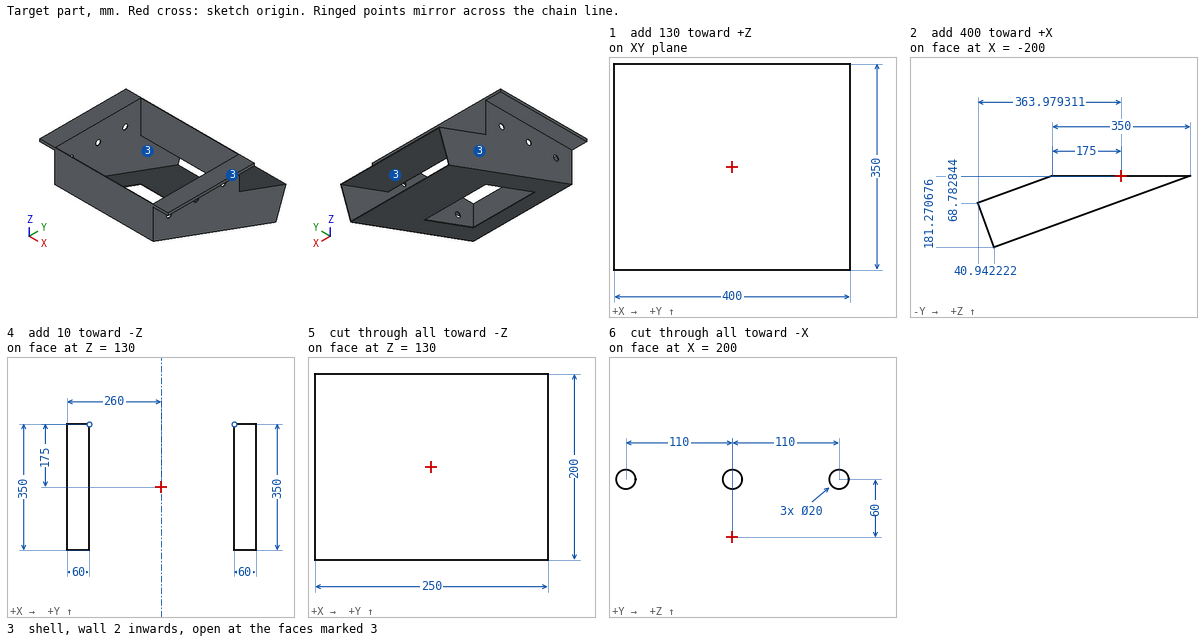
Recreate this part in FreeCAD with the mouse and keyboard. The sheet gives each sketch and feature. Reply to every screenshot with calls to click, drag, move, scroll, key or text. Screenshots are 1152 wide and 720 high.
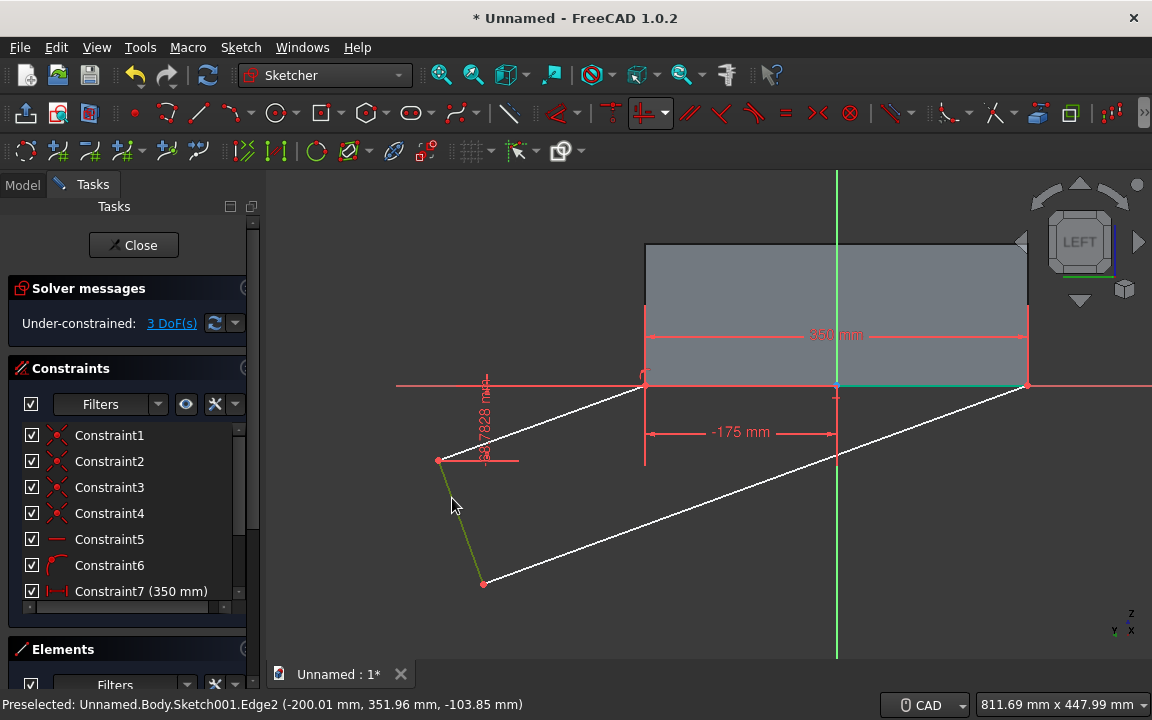
key(l)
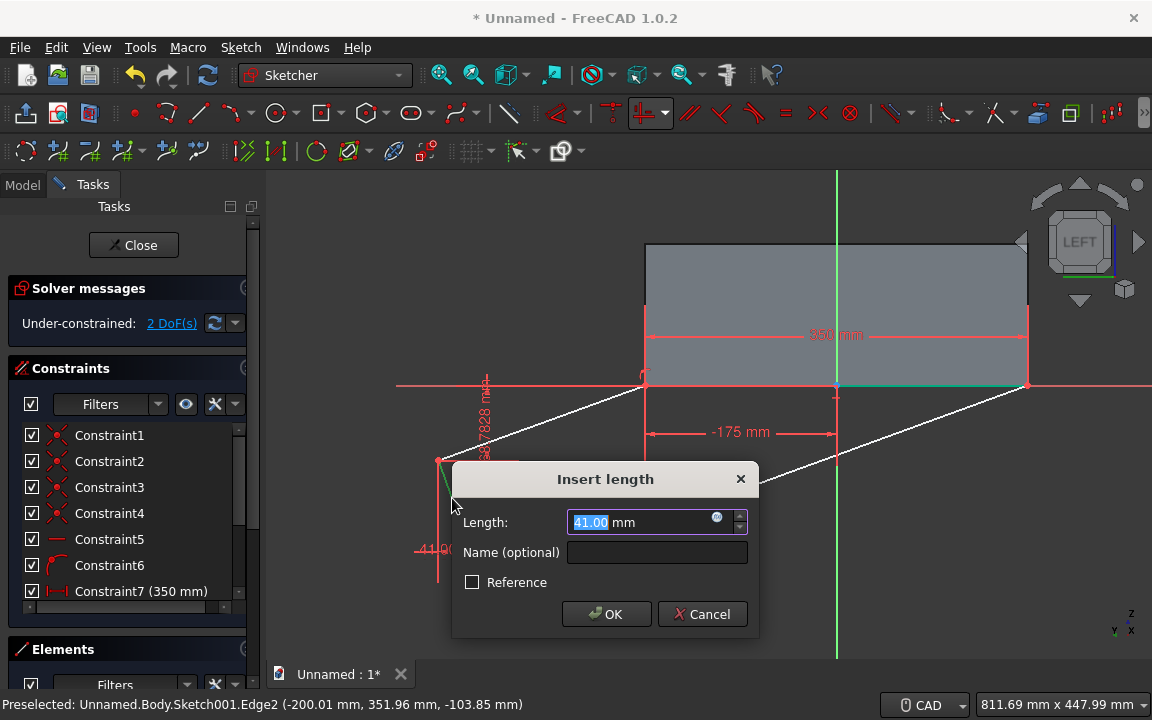
text(40.942222)
key(Return)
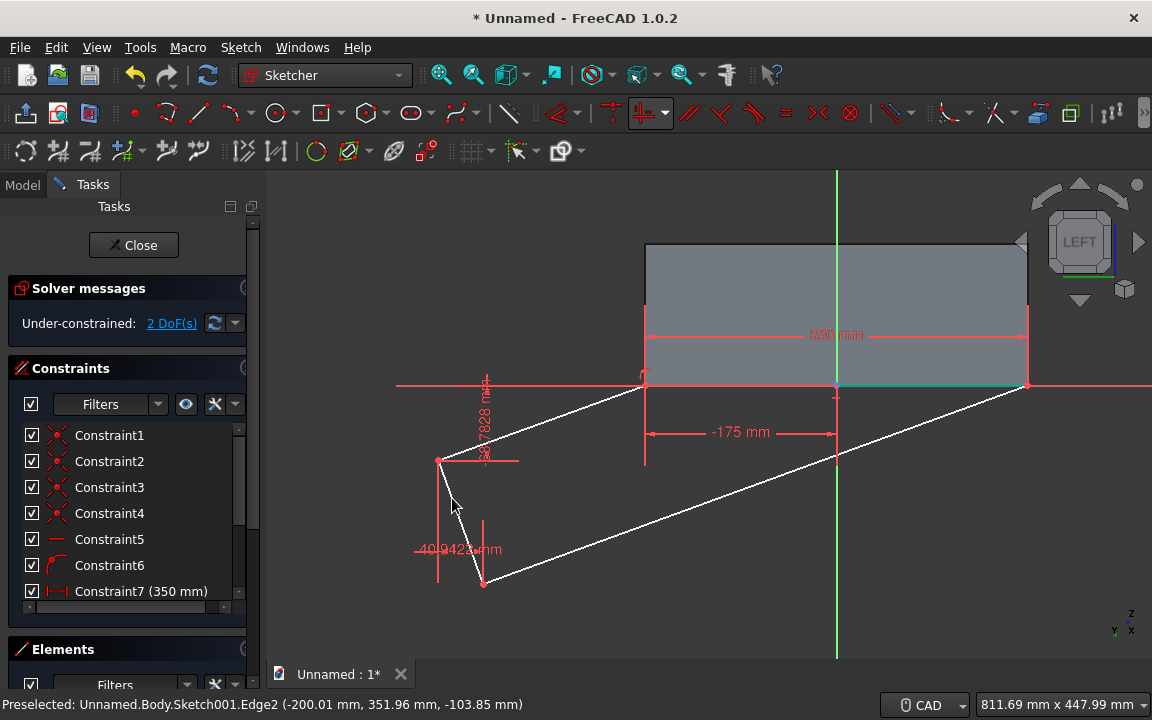
click(438, 461)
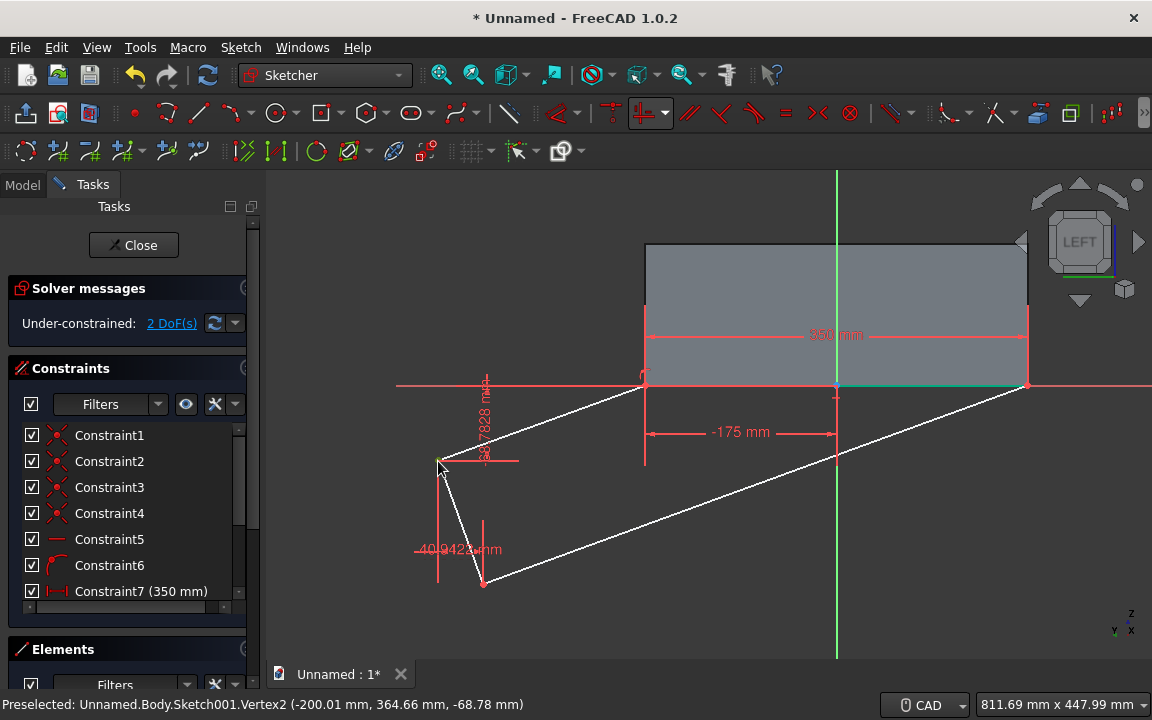
key(l)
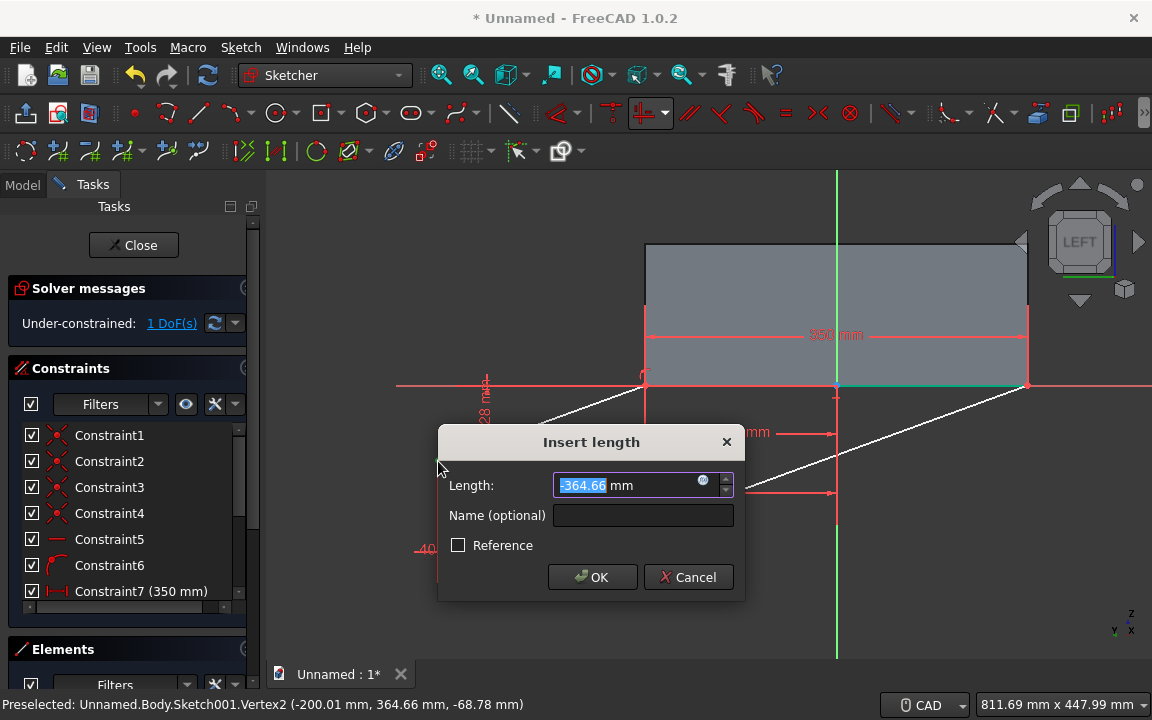
text(-363.979311)
key(Return)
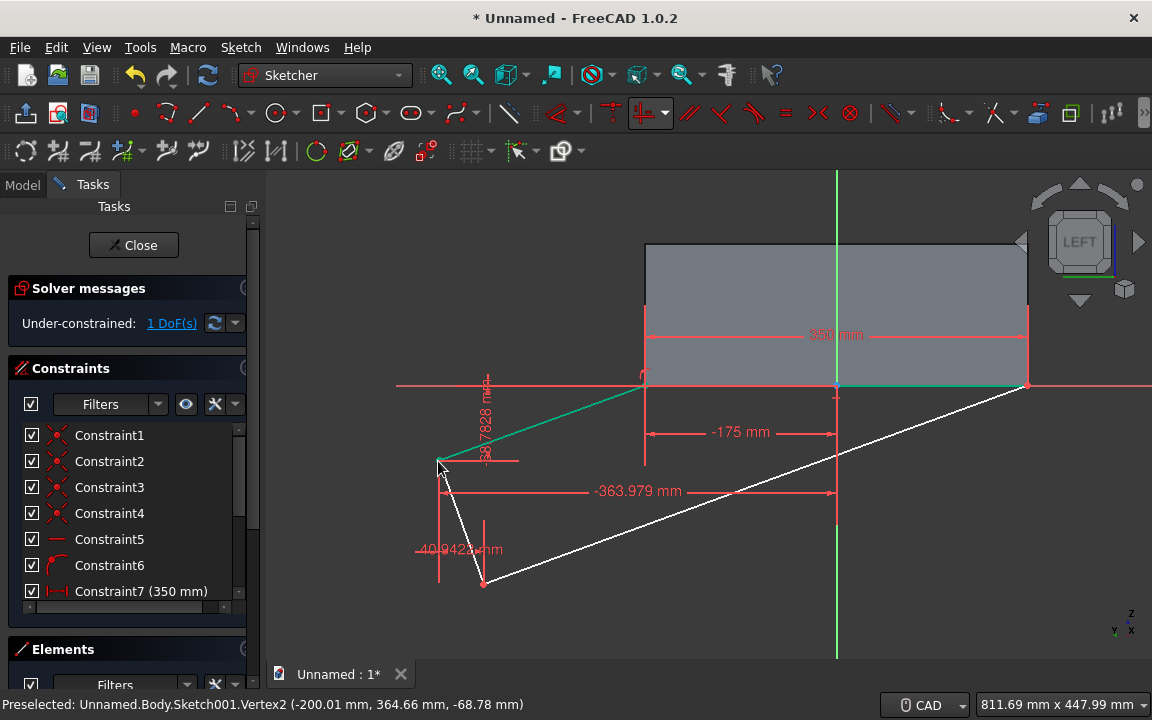
click(484, 584)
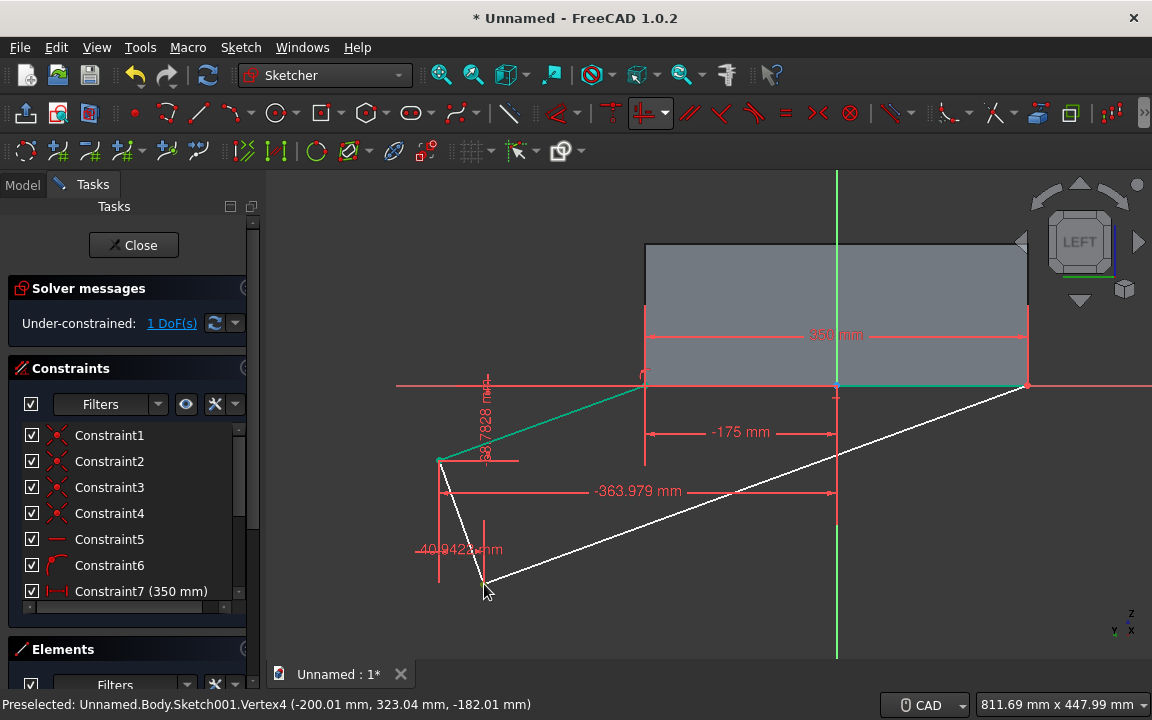
key(i)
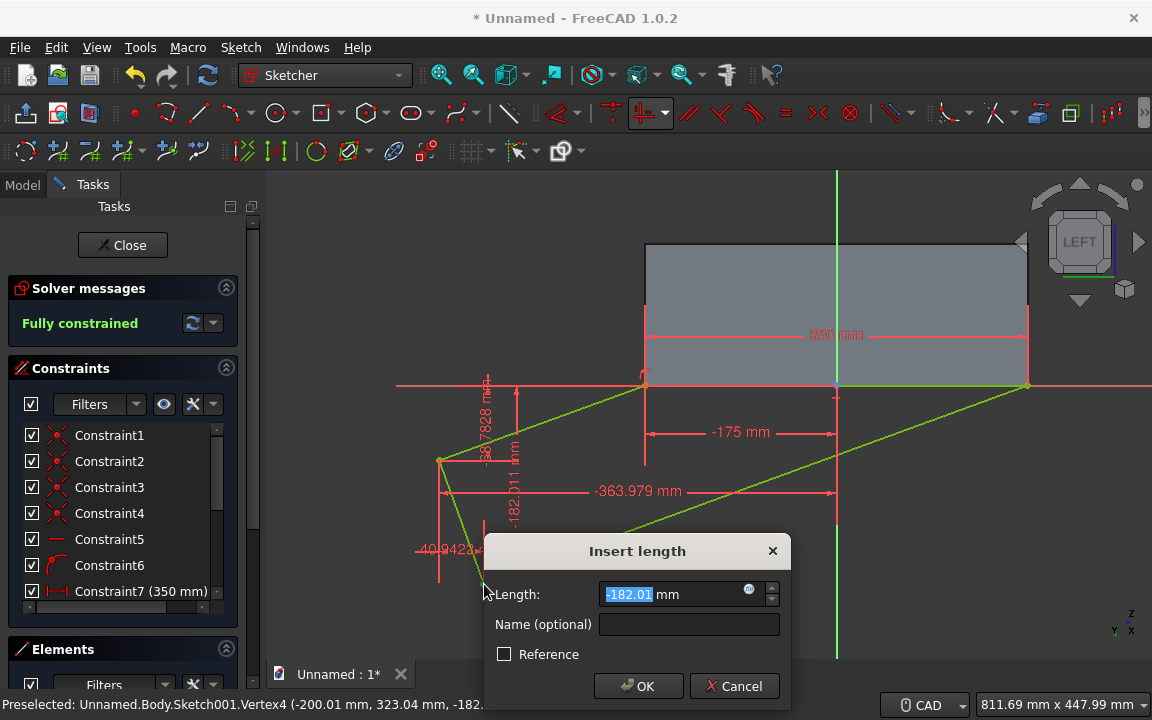
text(-181.270676)
key(Return)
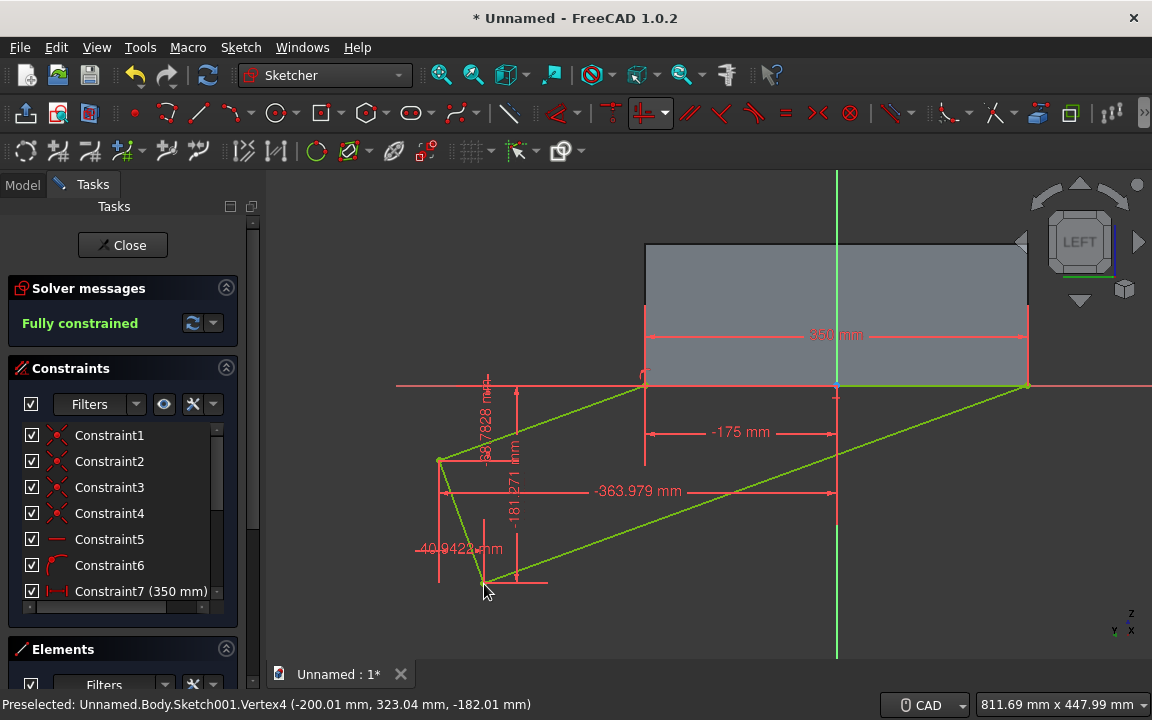
click(123, 245)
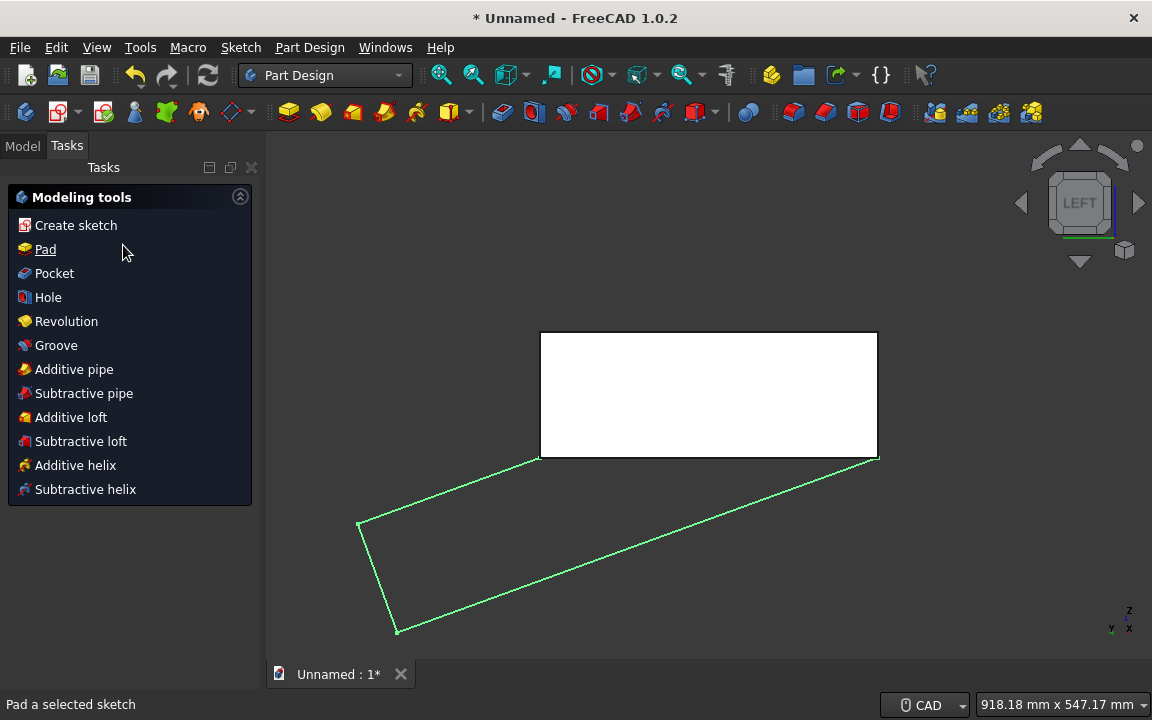
click(290, 112)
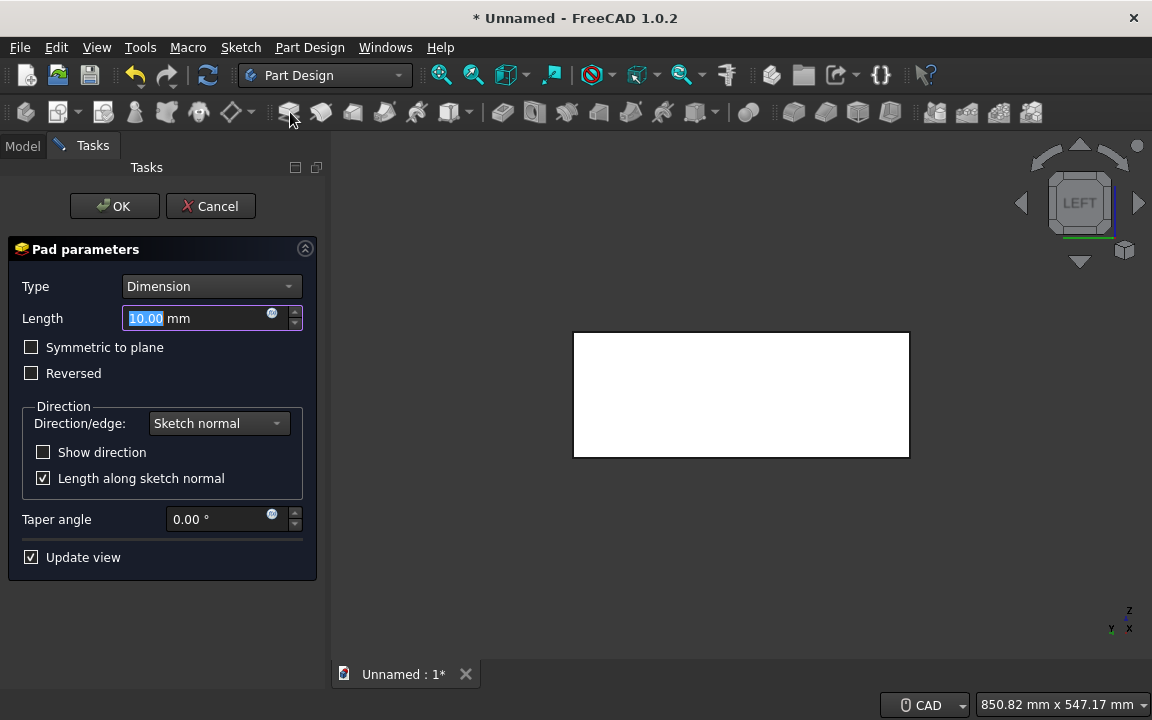
text(400)
key(Tab)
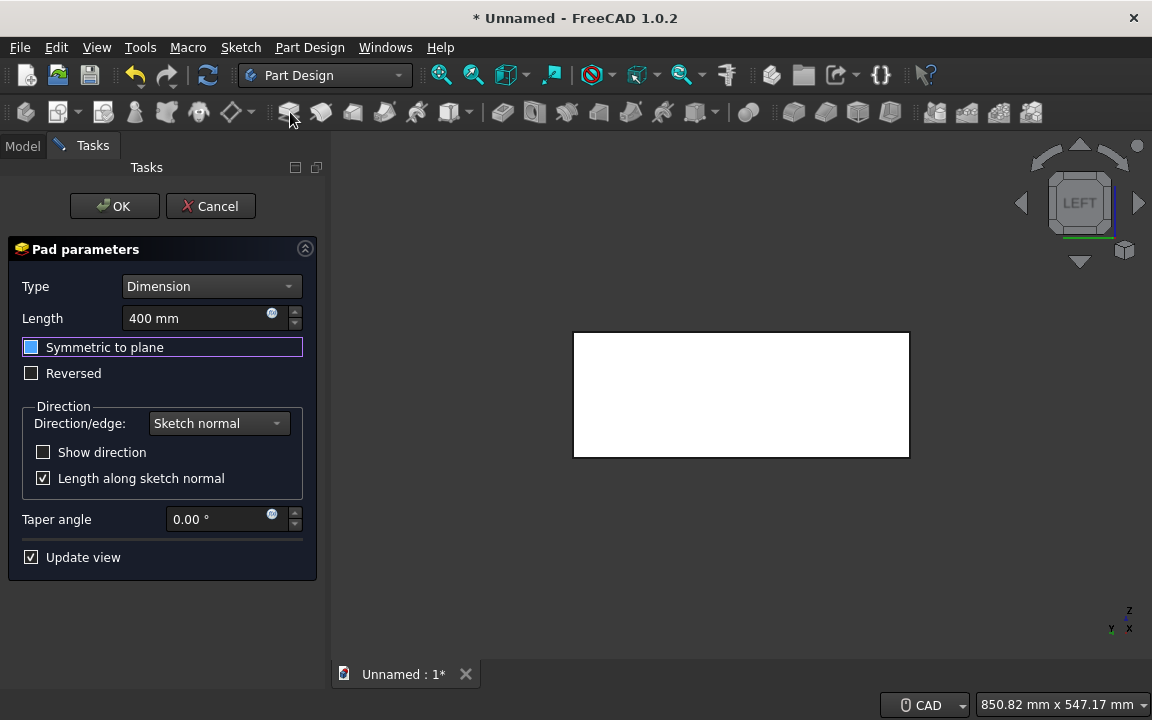
click(30, 373)